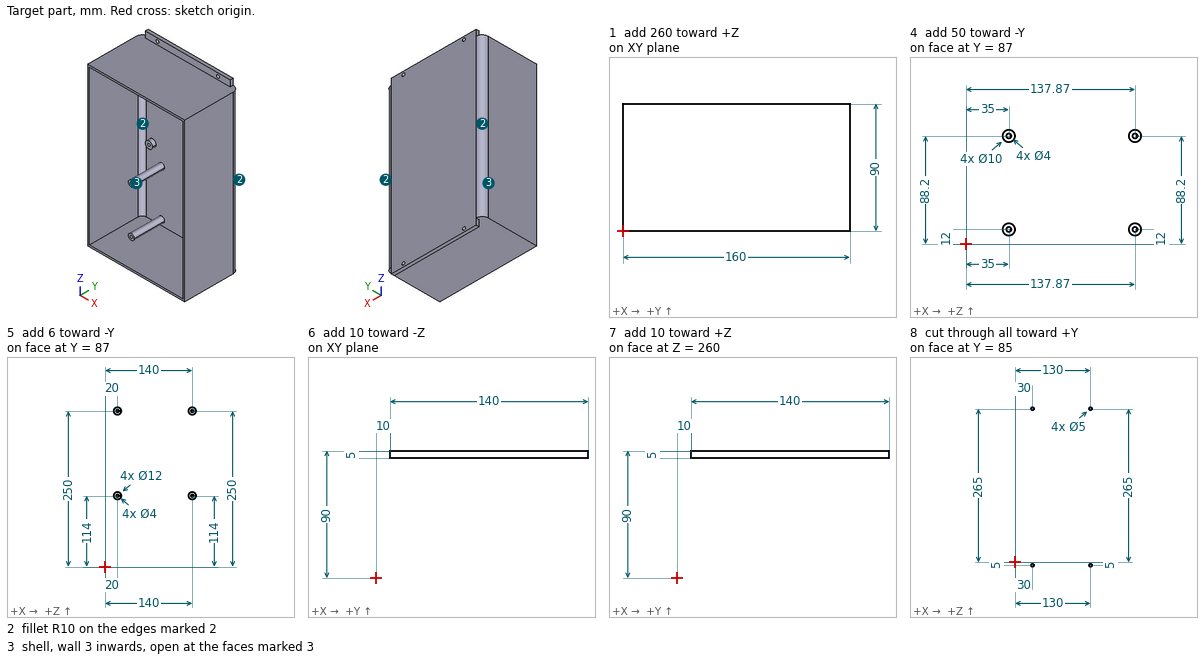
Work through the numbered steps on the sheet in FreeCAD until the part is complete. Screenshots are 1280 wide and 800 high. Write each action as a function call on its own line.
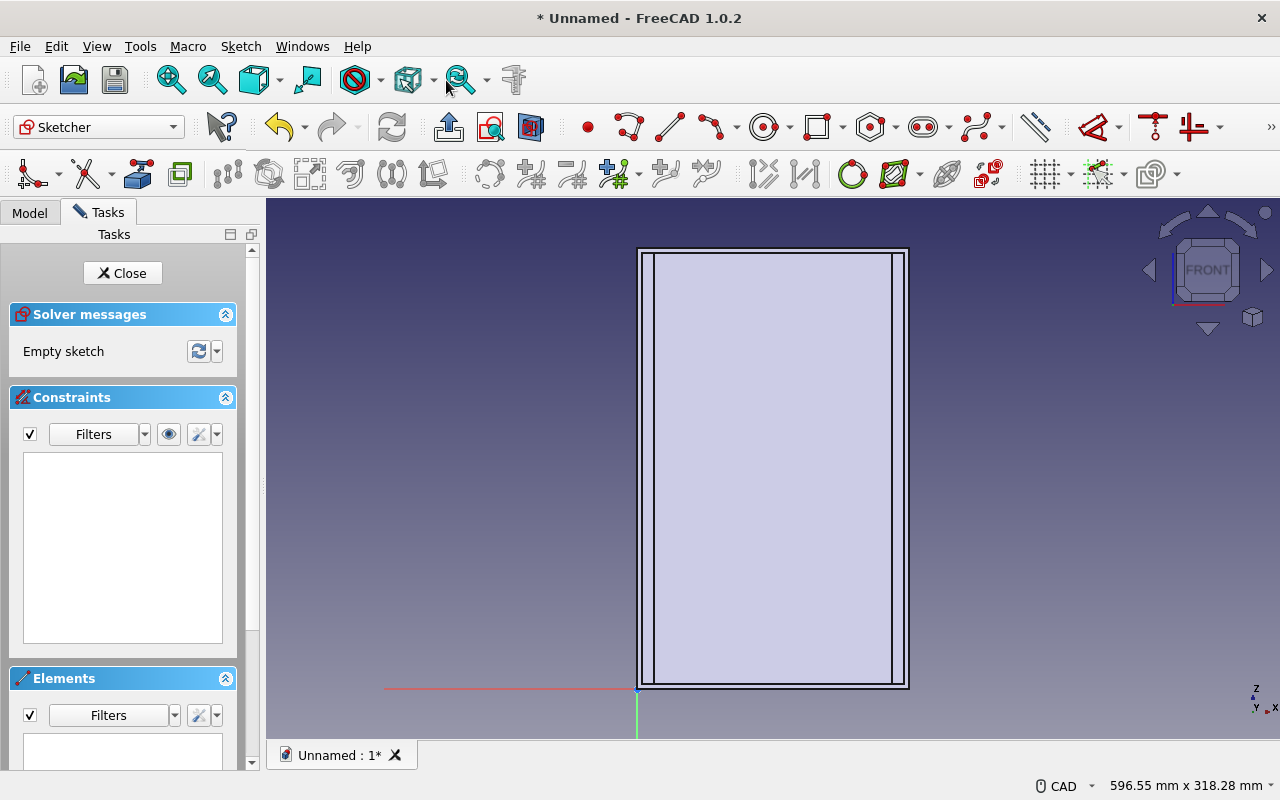
click(531, 128)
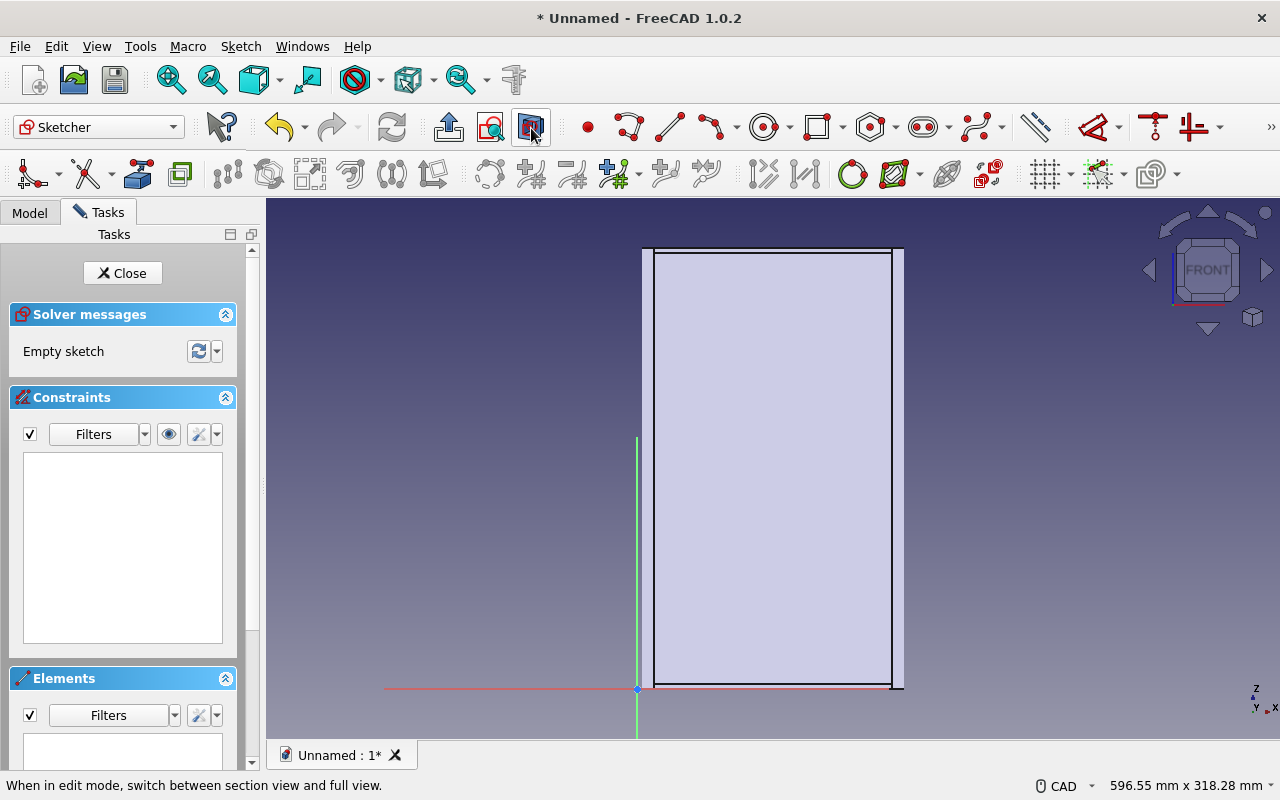
scroll(802, 711, up, 4)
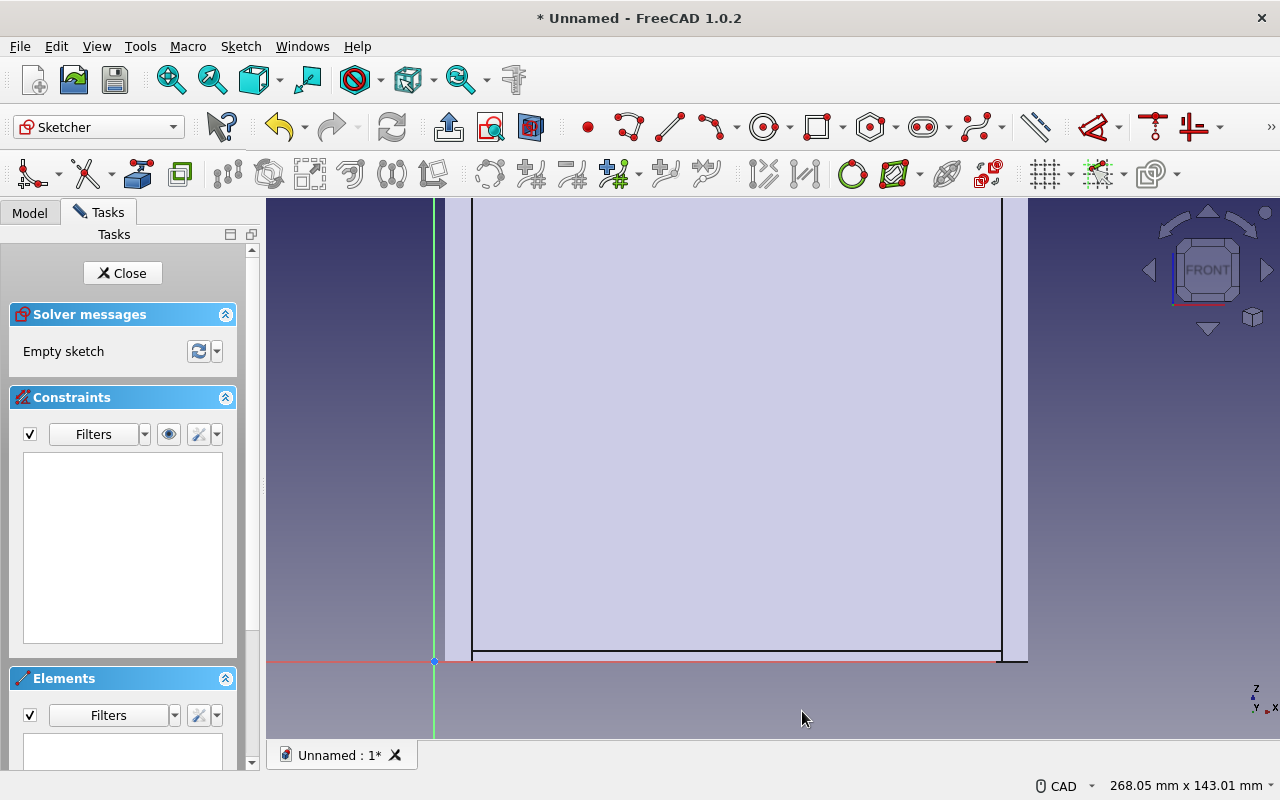
click(764, 128)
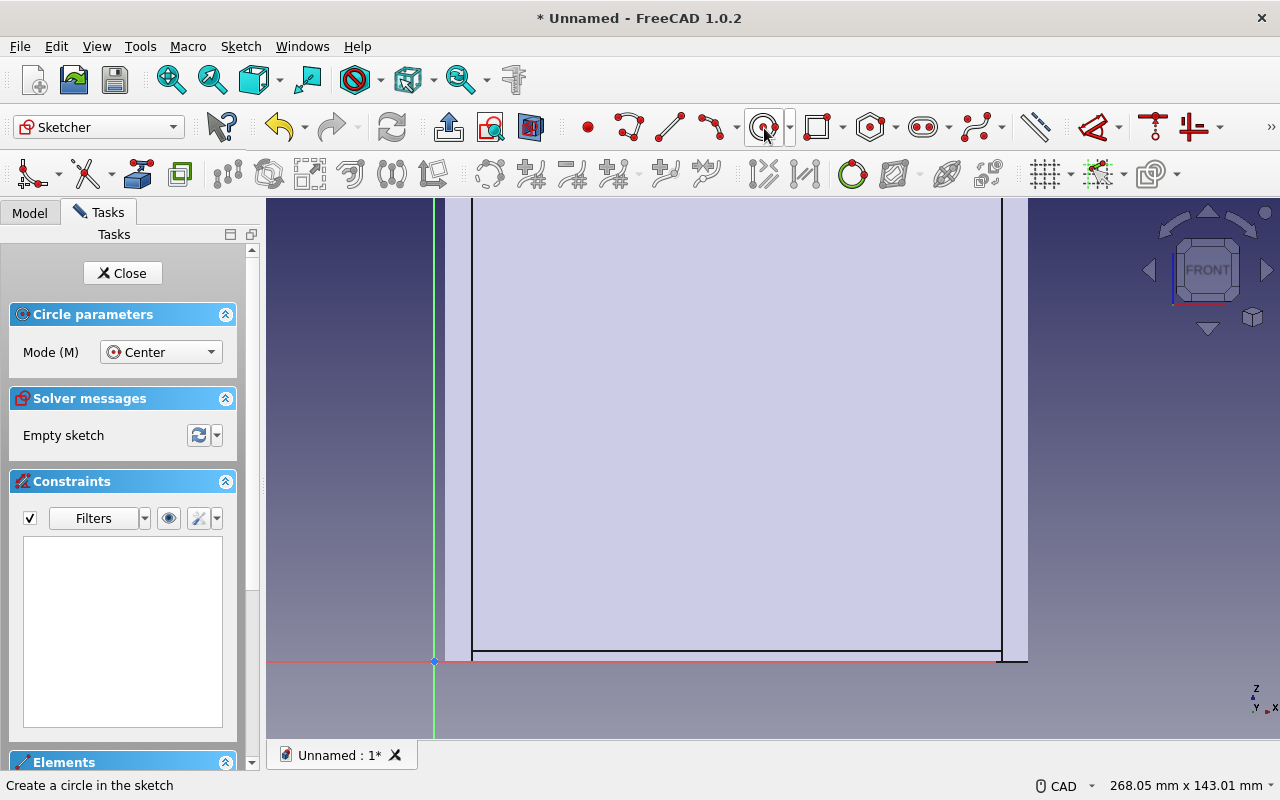
click(567, 328)
click(580, 315)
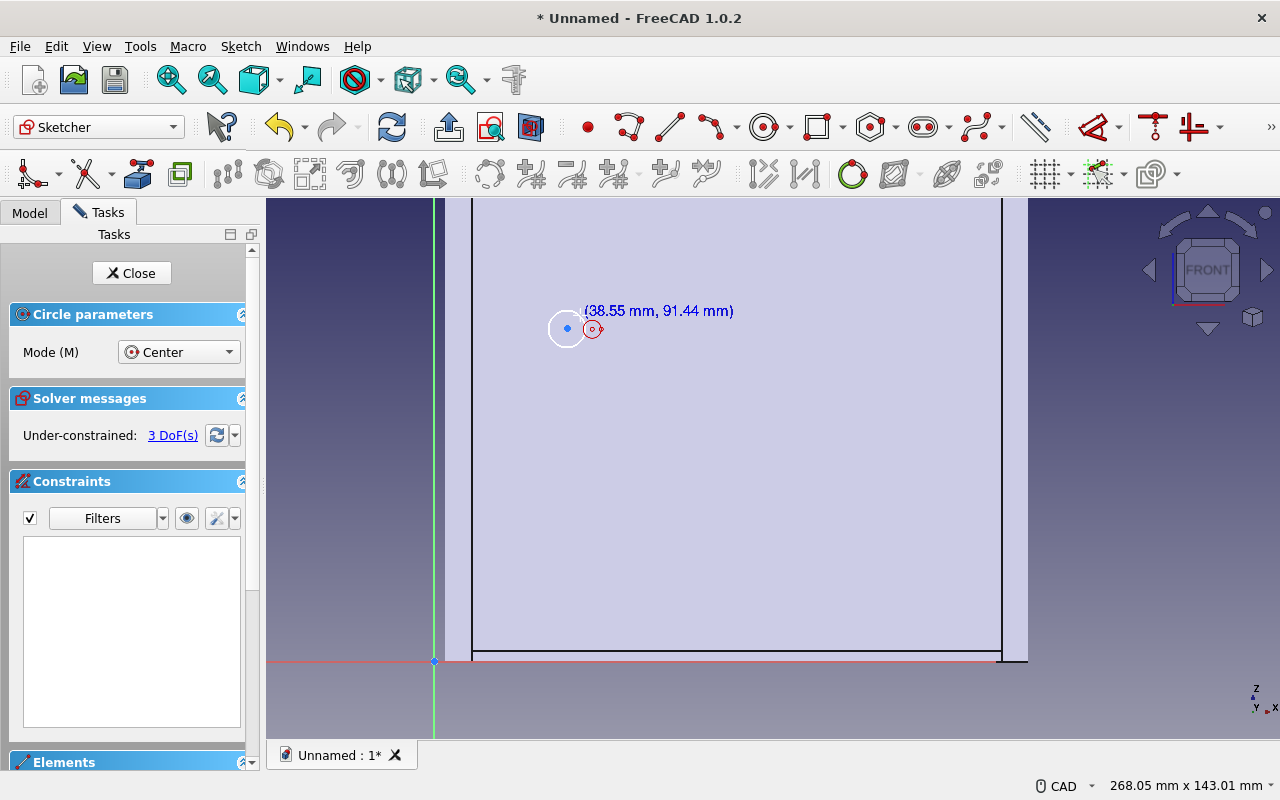
click(567, 617)
click(580, 603)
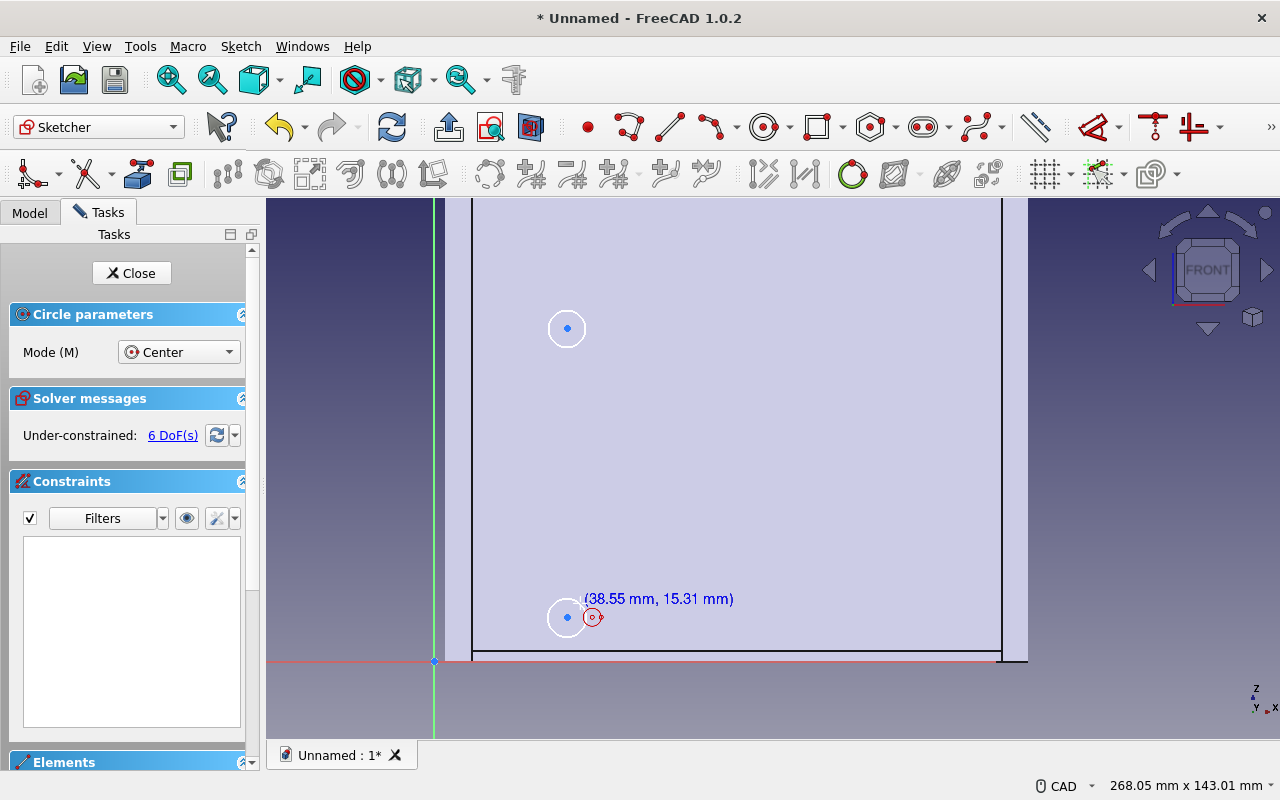
click(956, 617)
click(969, 603)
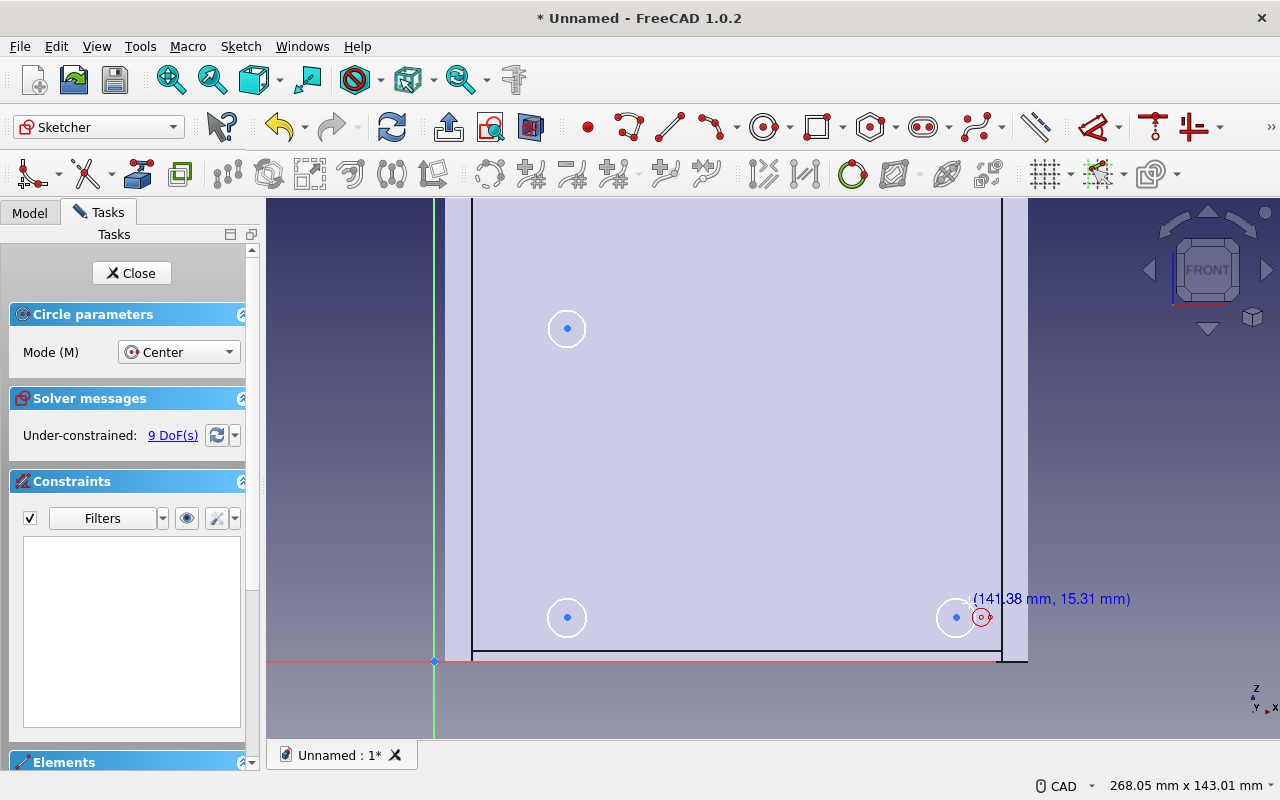
click(956, 328)
click(969, 315)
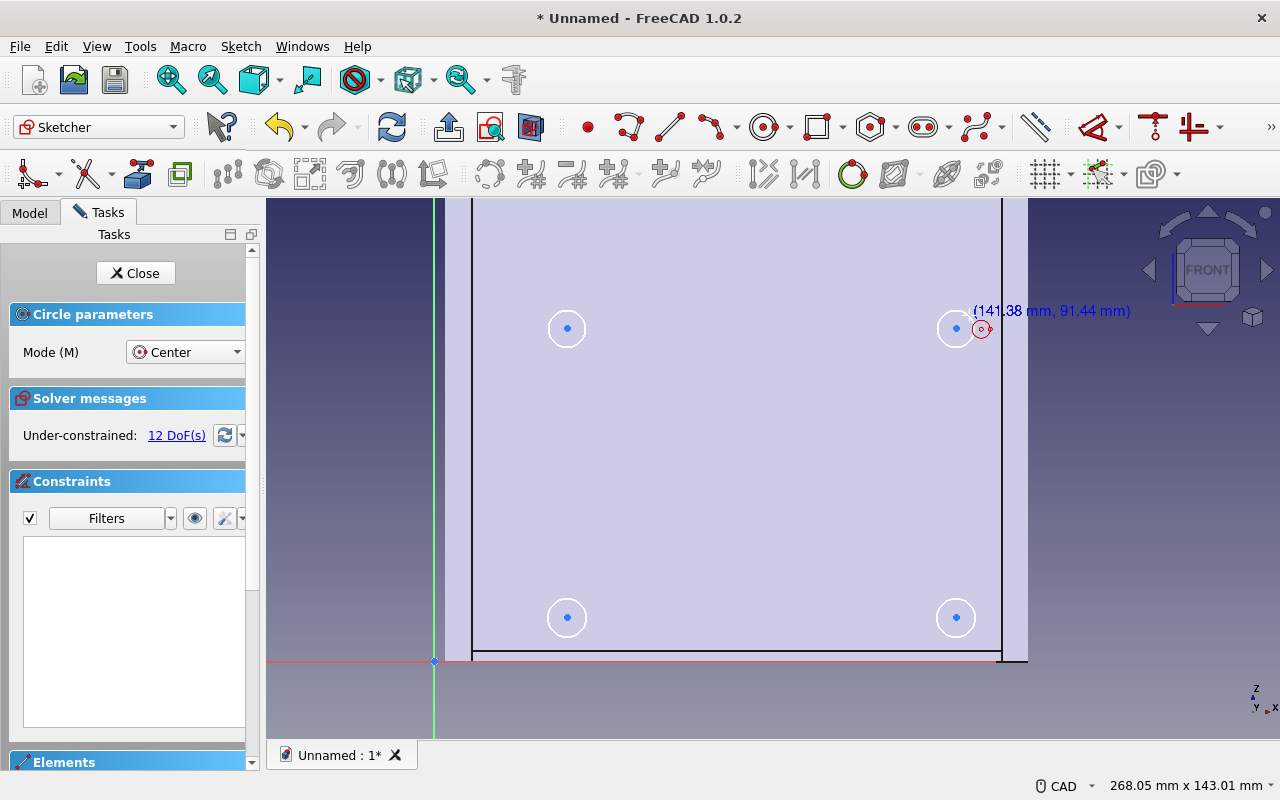
scroll(567, 328, up, 6)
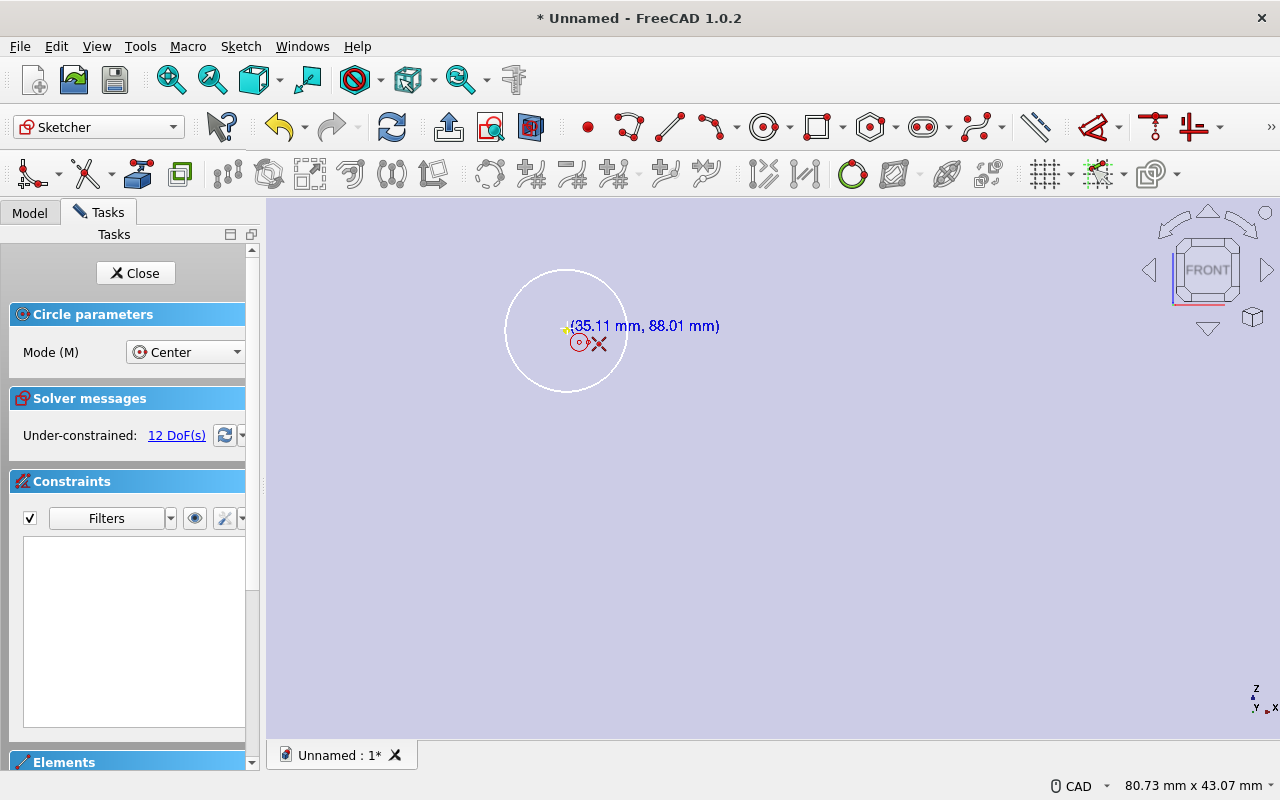
click(566, 331)
click(583, 311)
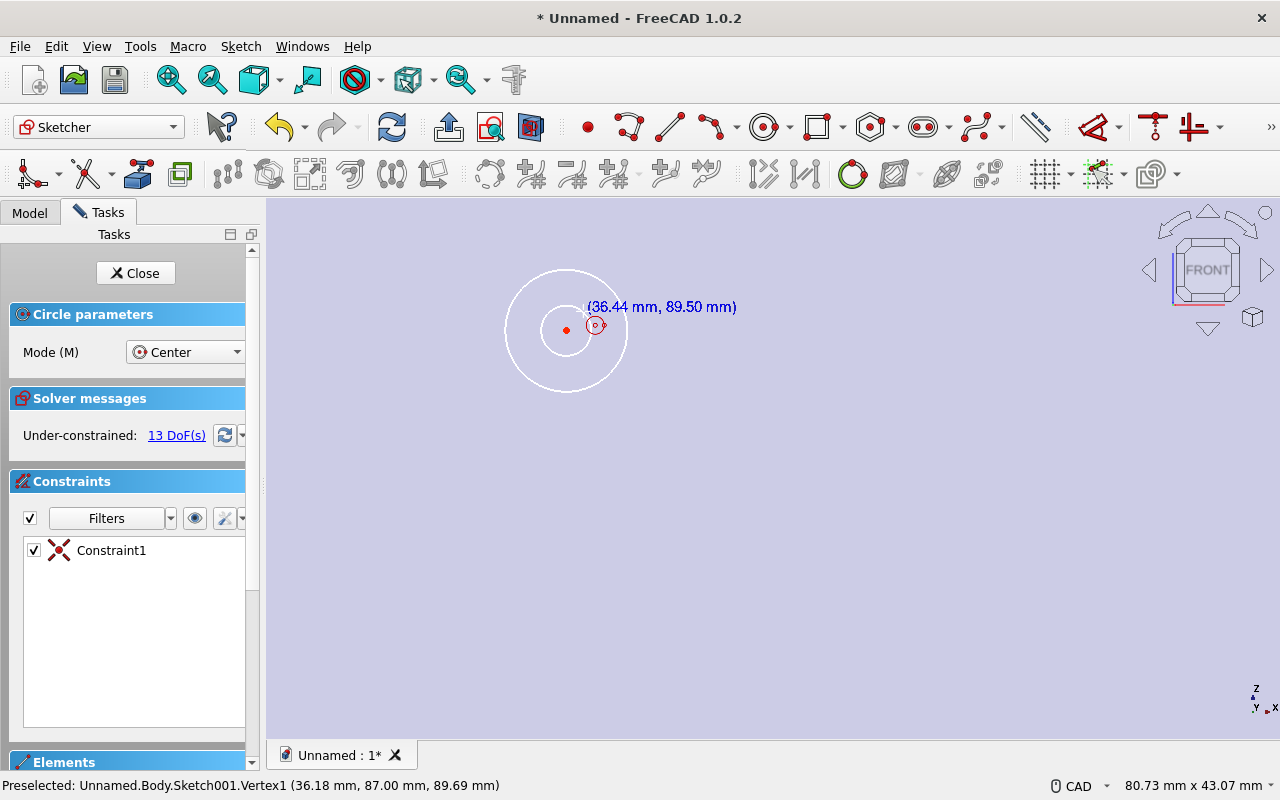
scroll(567, 304, down, 6)